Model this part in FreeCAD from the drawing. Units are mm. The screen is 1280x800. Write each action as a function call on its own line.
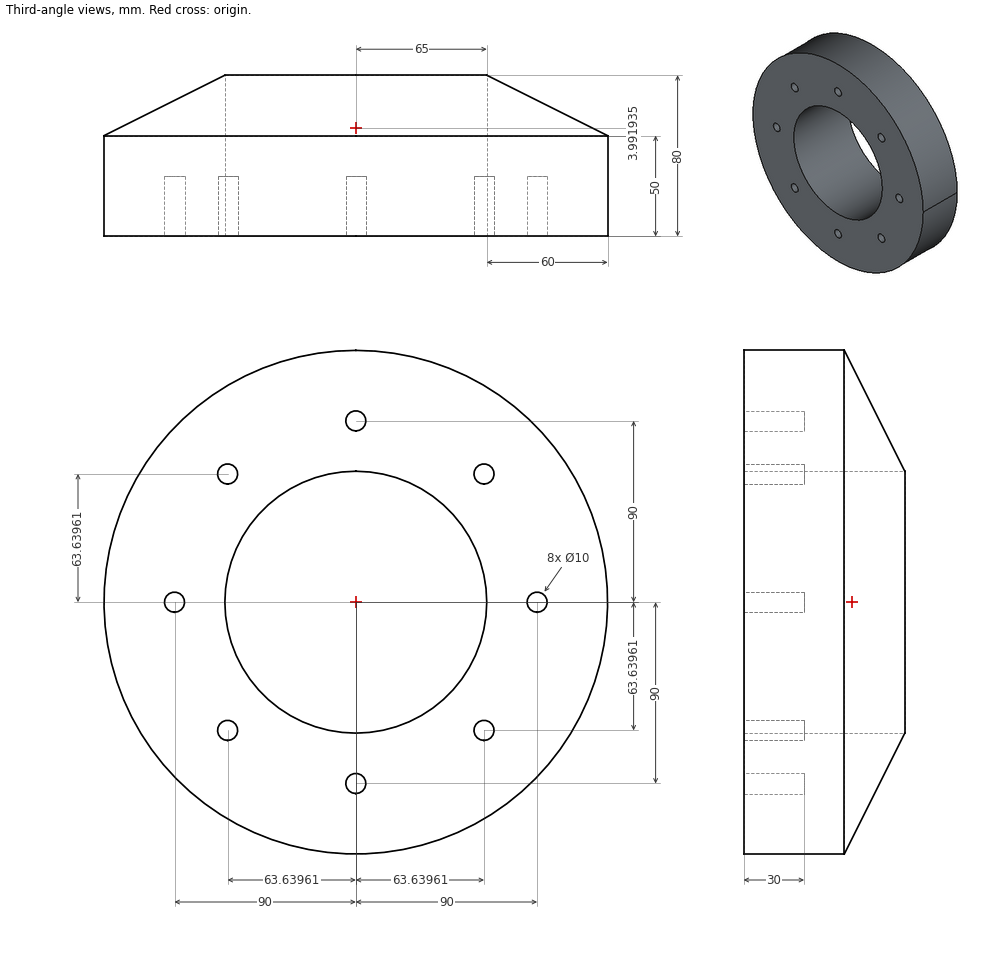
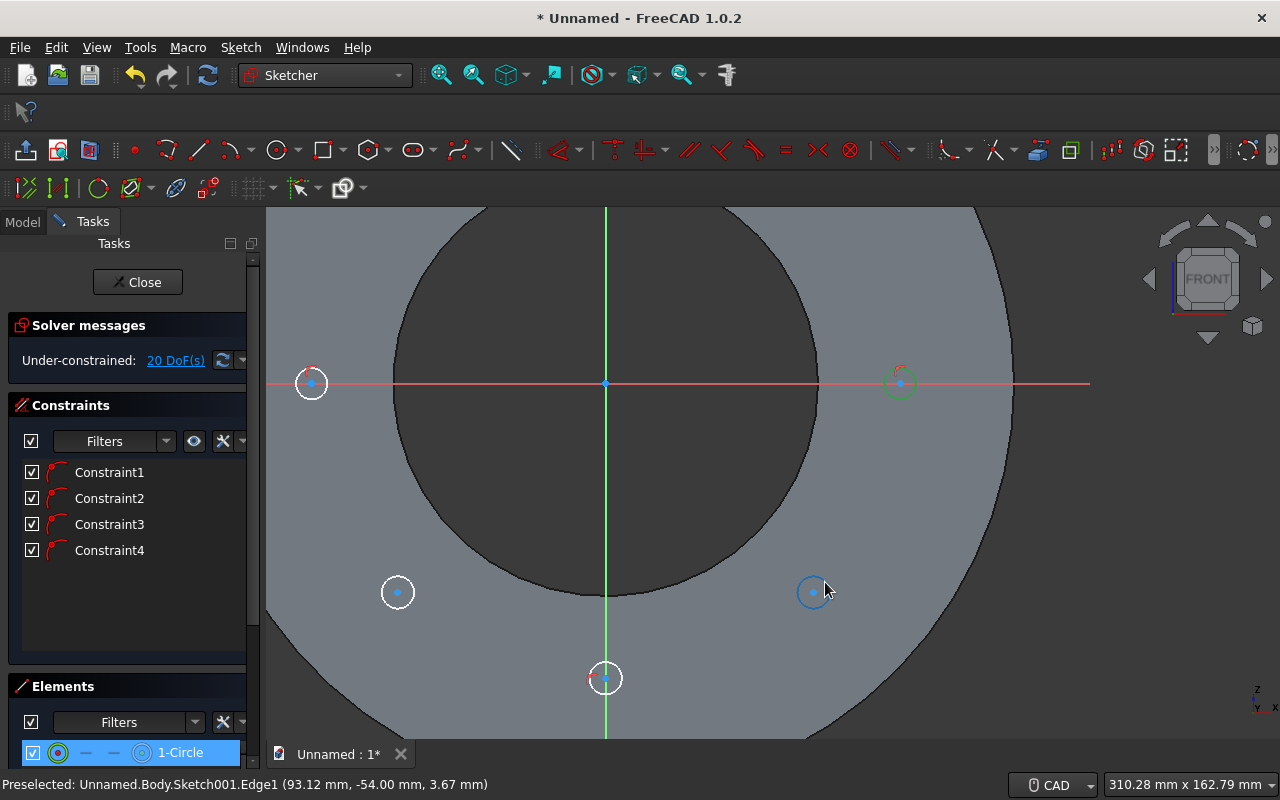
click(825, 581)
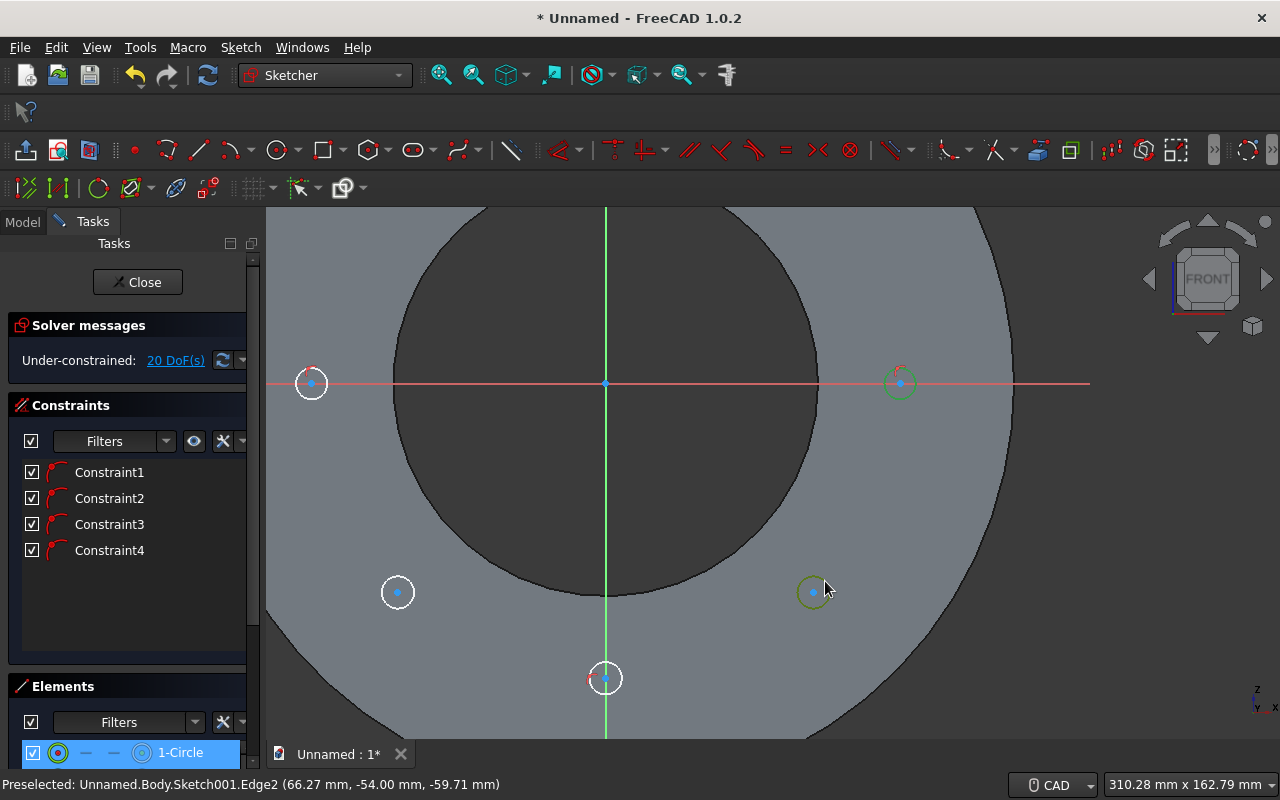
click(617, 667)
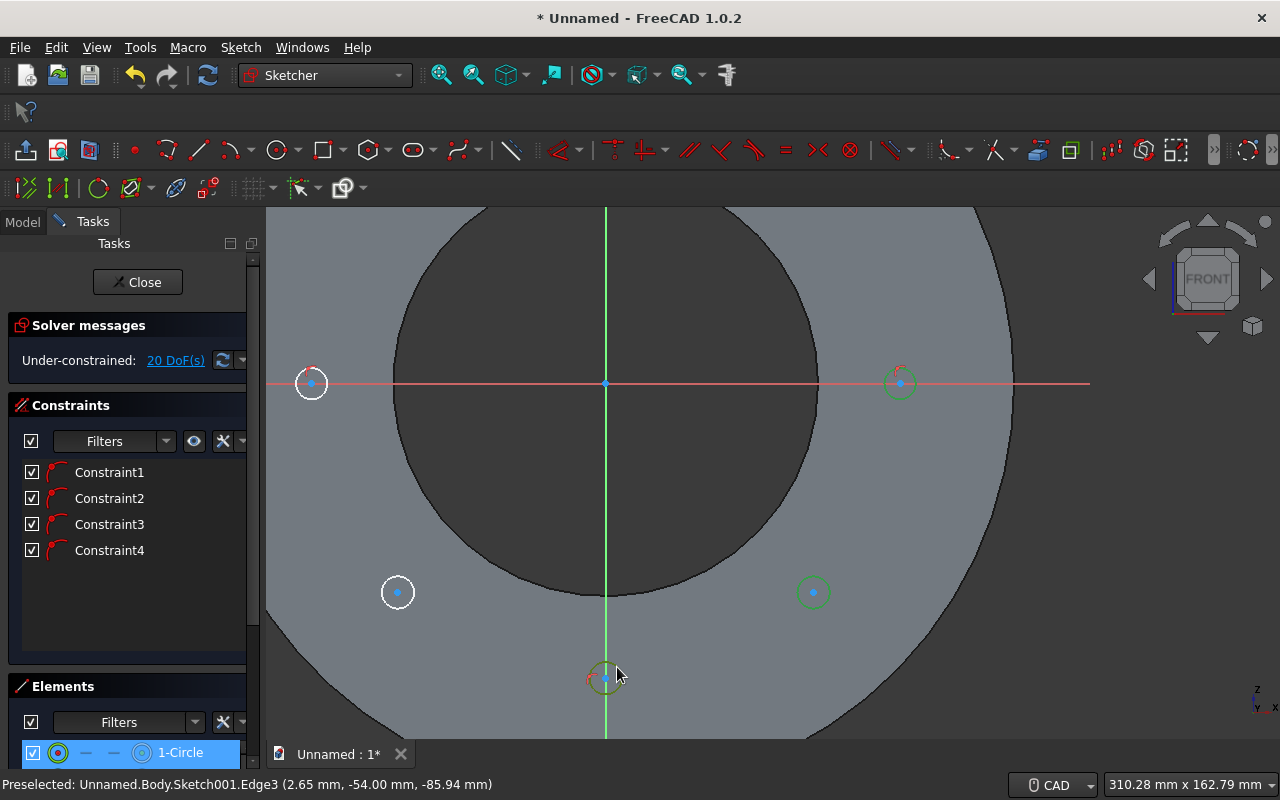
click(409, 581)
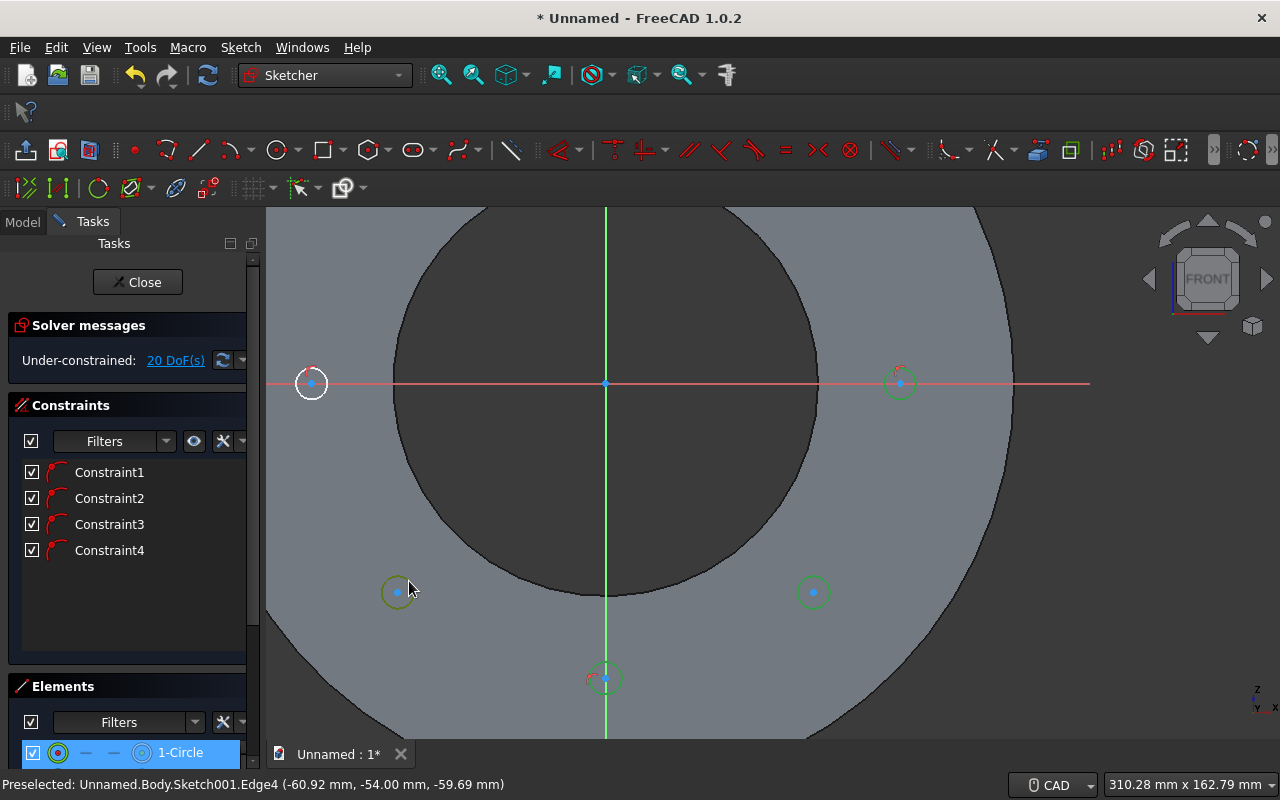
scroll(323, 373, up, 2)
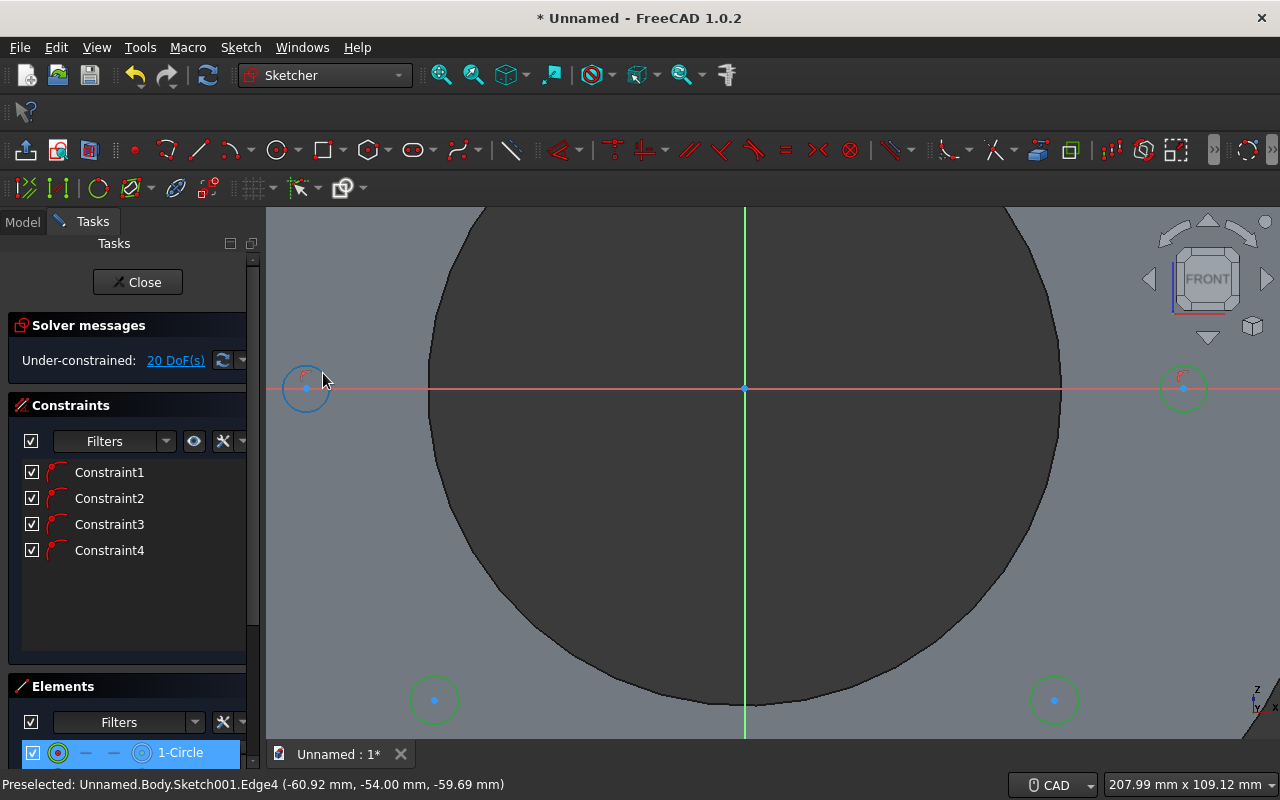
click(322, 372)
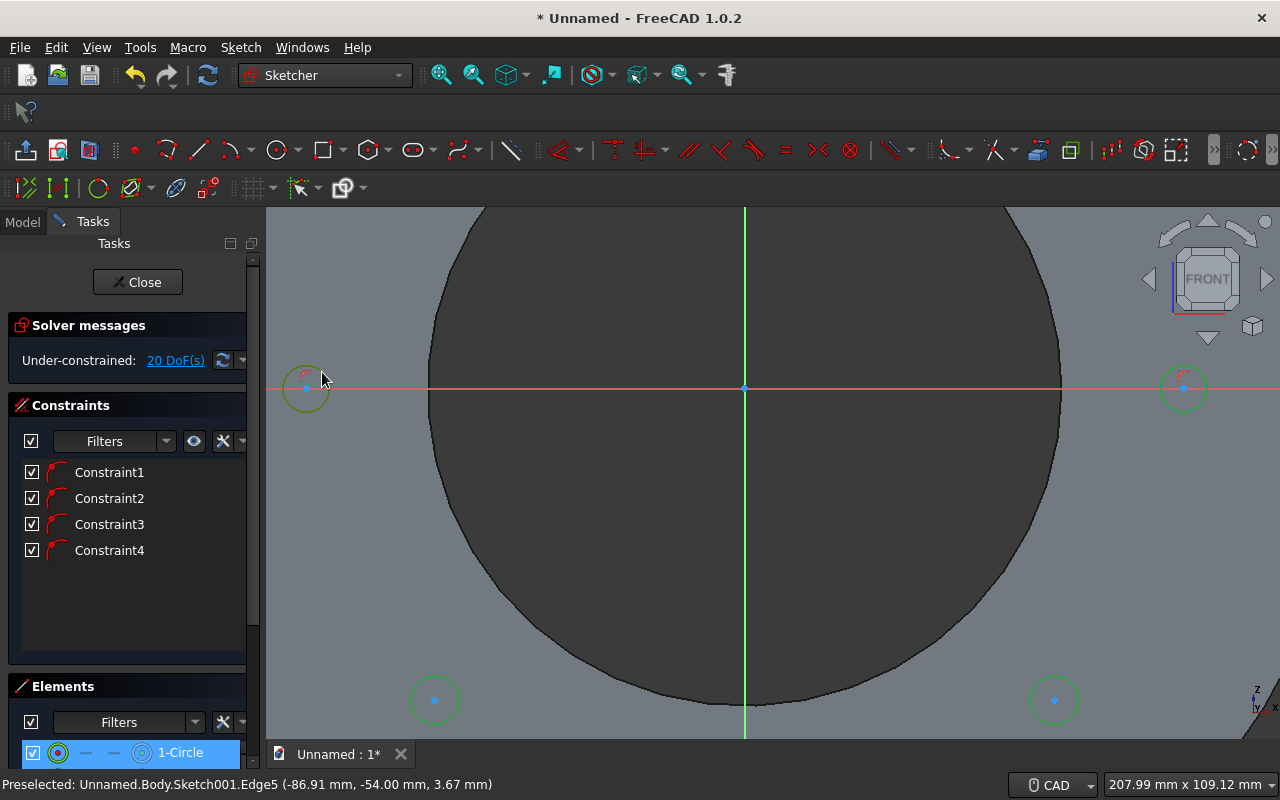
scroll(681, 522, down, 5)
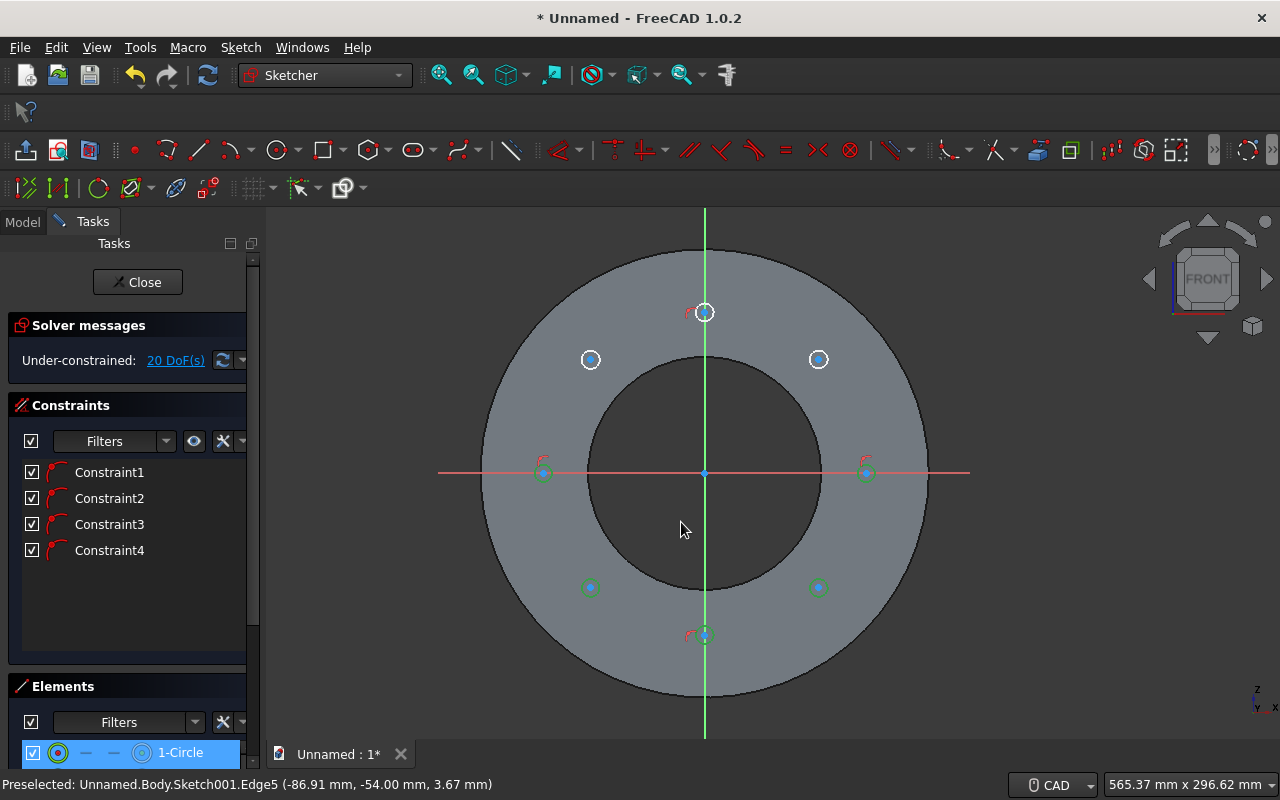
scroll(597, 353, up, 3)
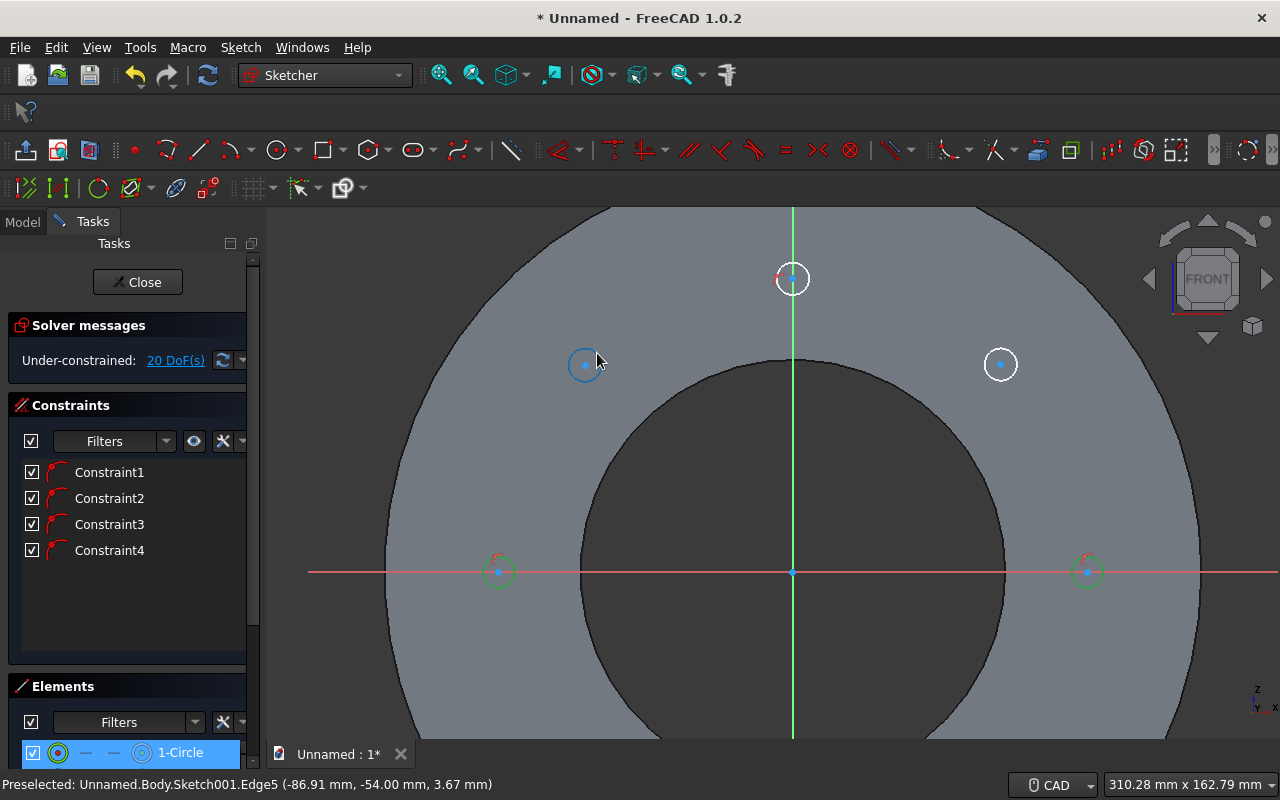
click(597, 353)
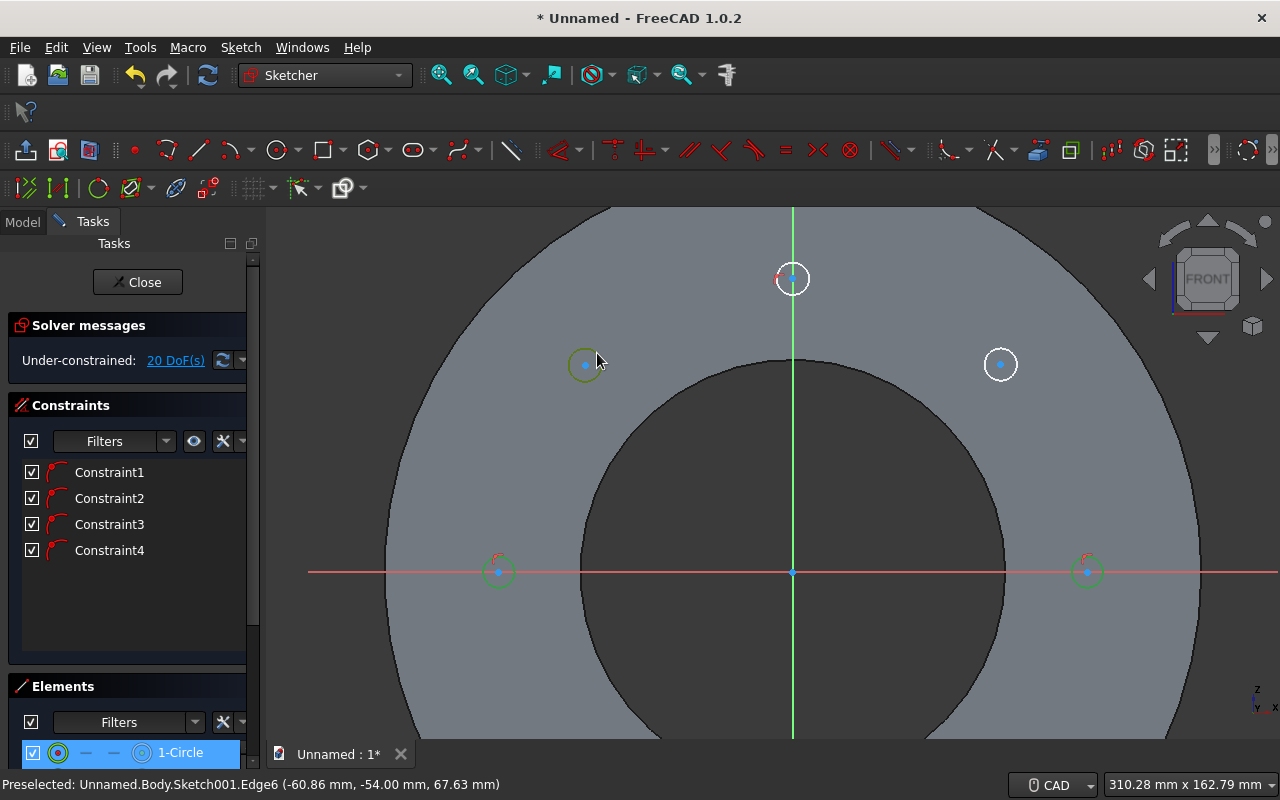
click(804, 267)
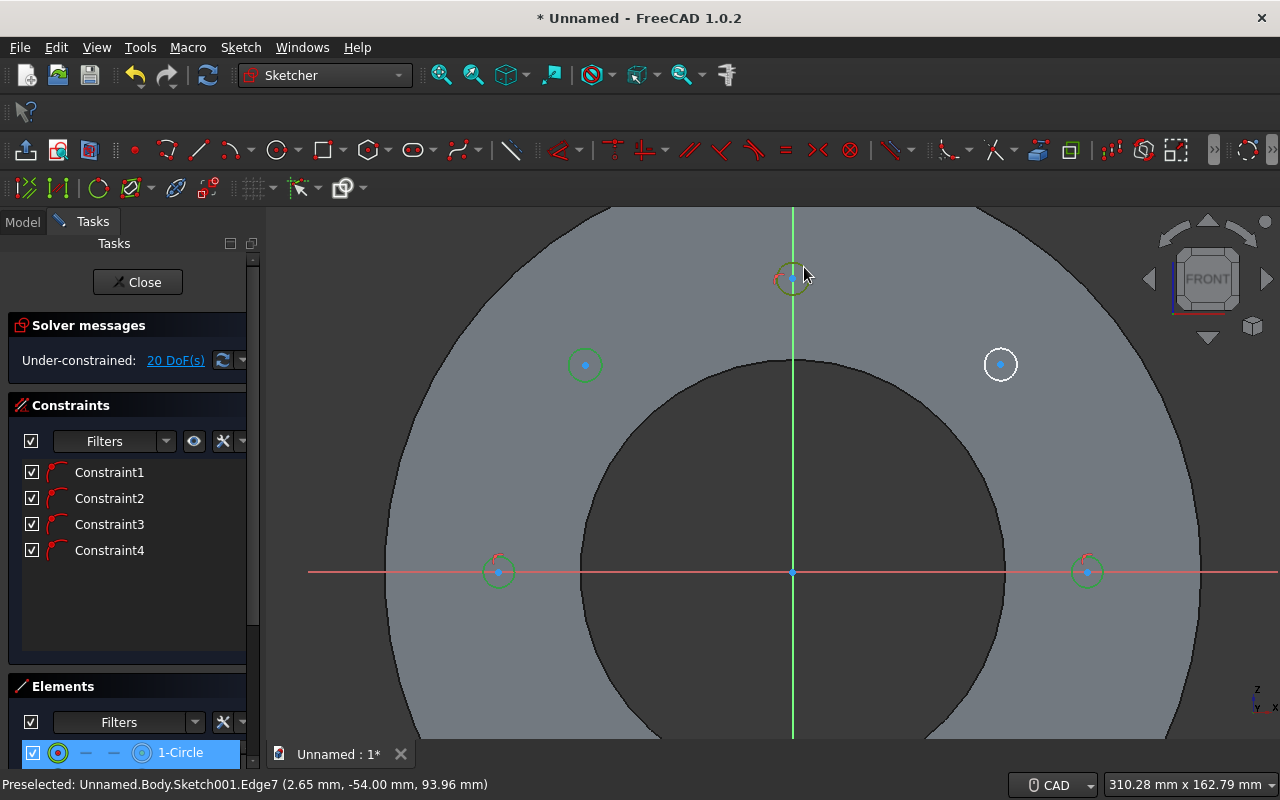
click(1012, 353)